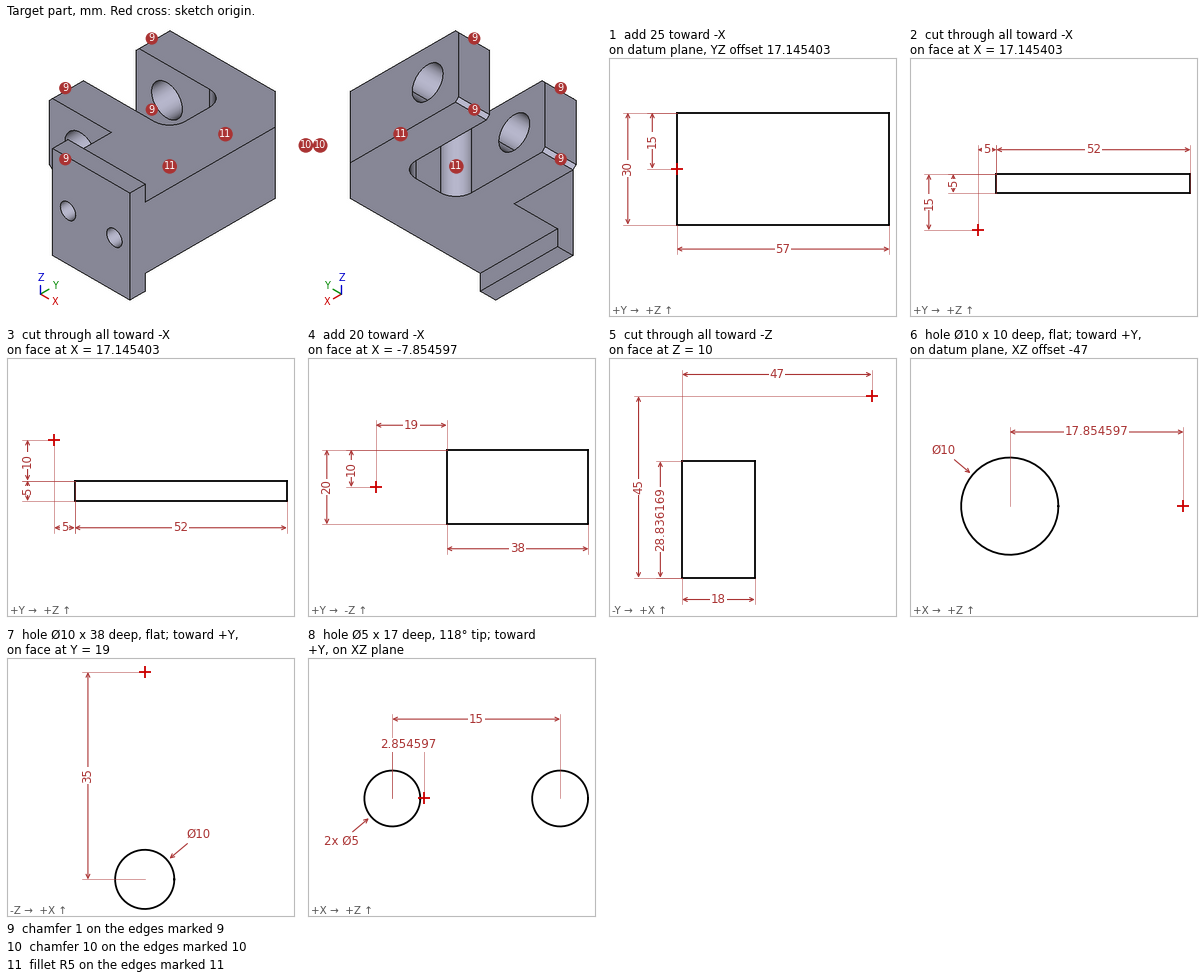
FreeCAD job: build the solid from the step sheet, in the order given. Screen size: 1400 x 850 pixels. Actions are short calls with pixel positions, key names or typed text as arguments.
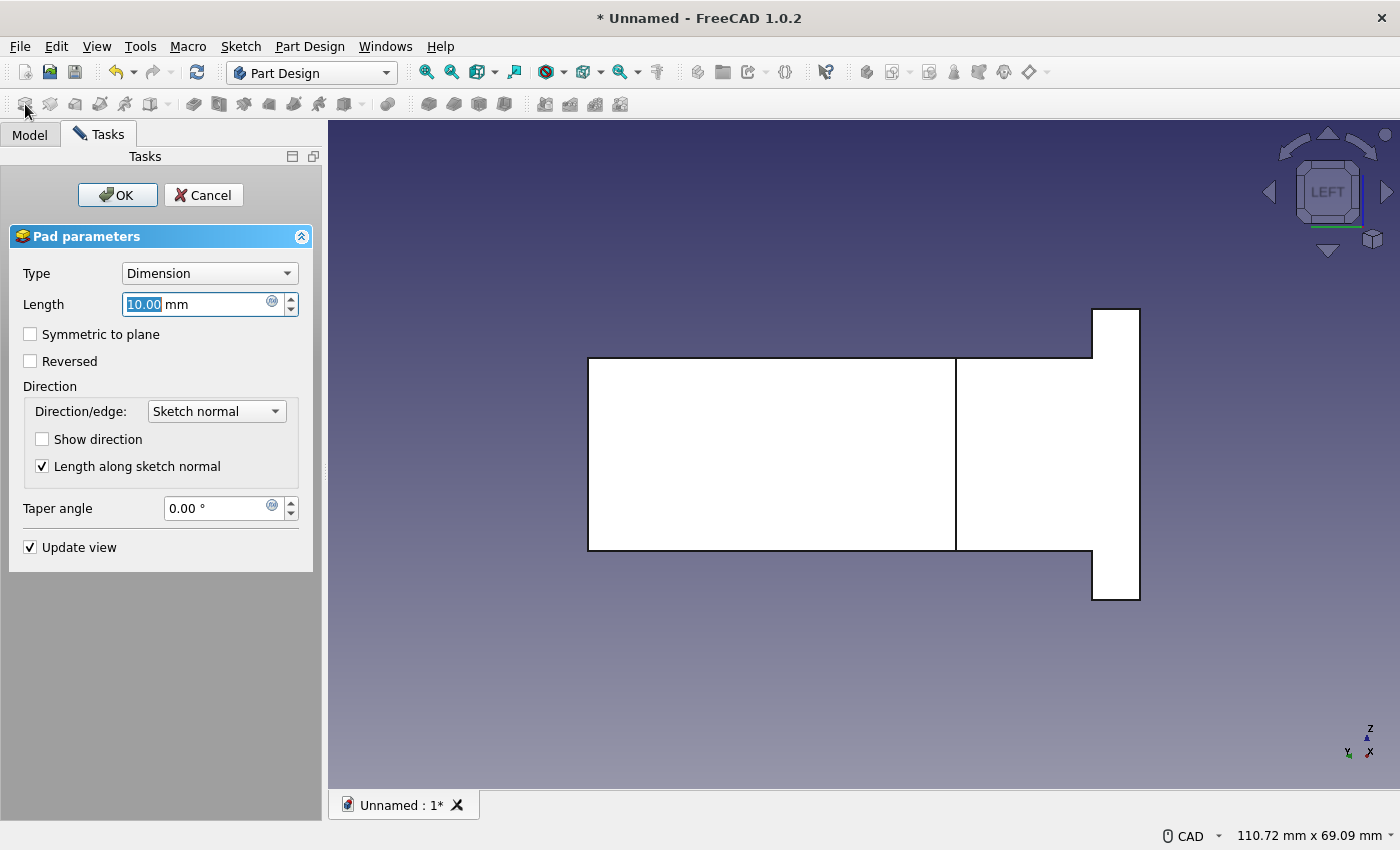
text(20)
key(Tab)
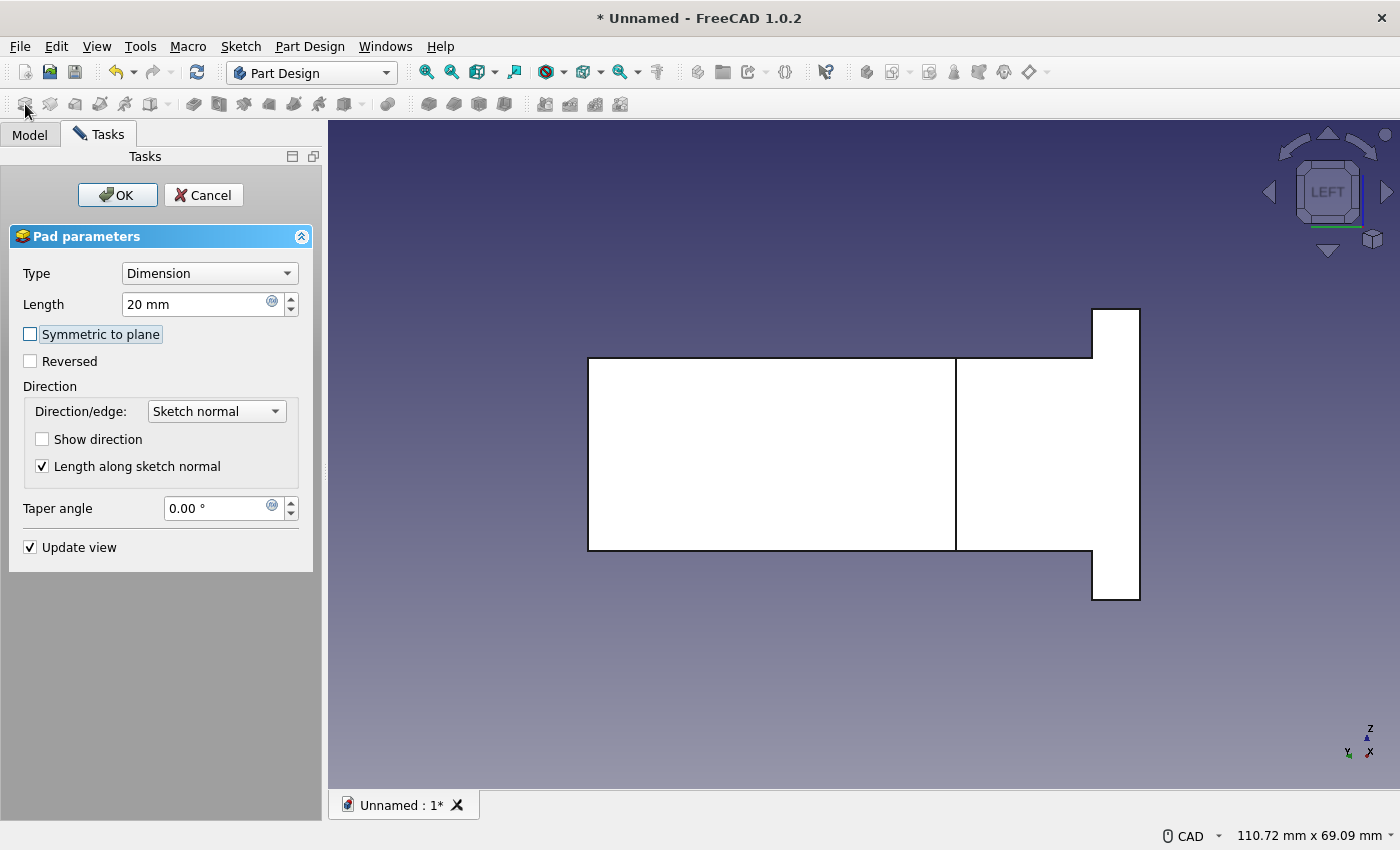
click(118, 195)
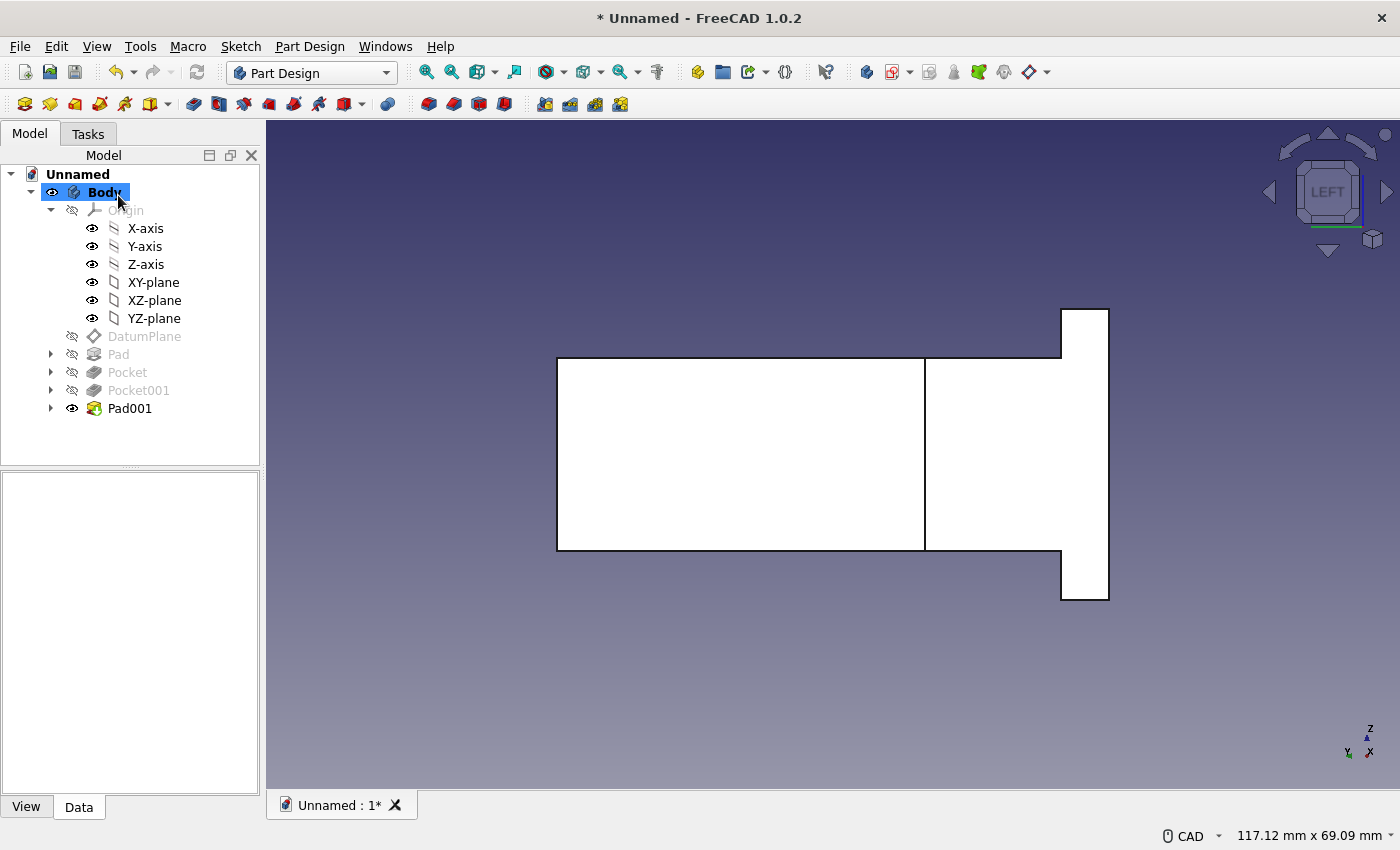
key(0)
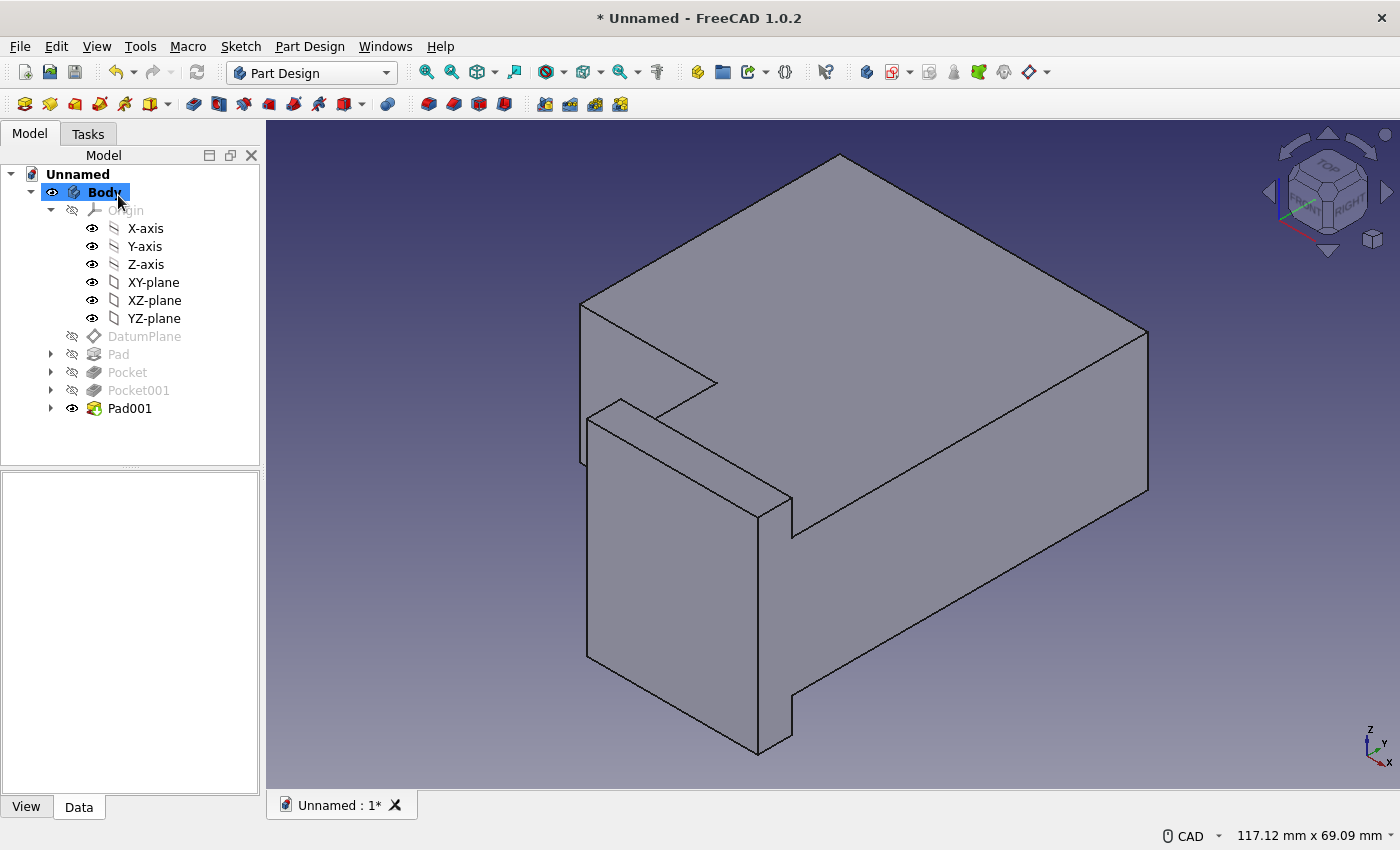
click(427, 72)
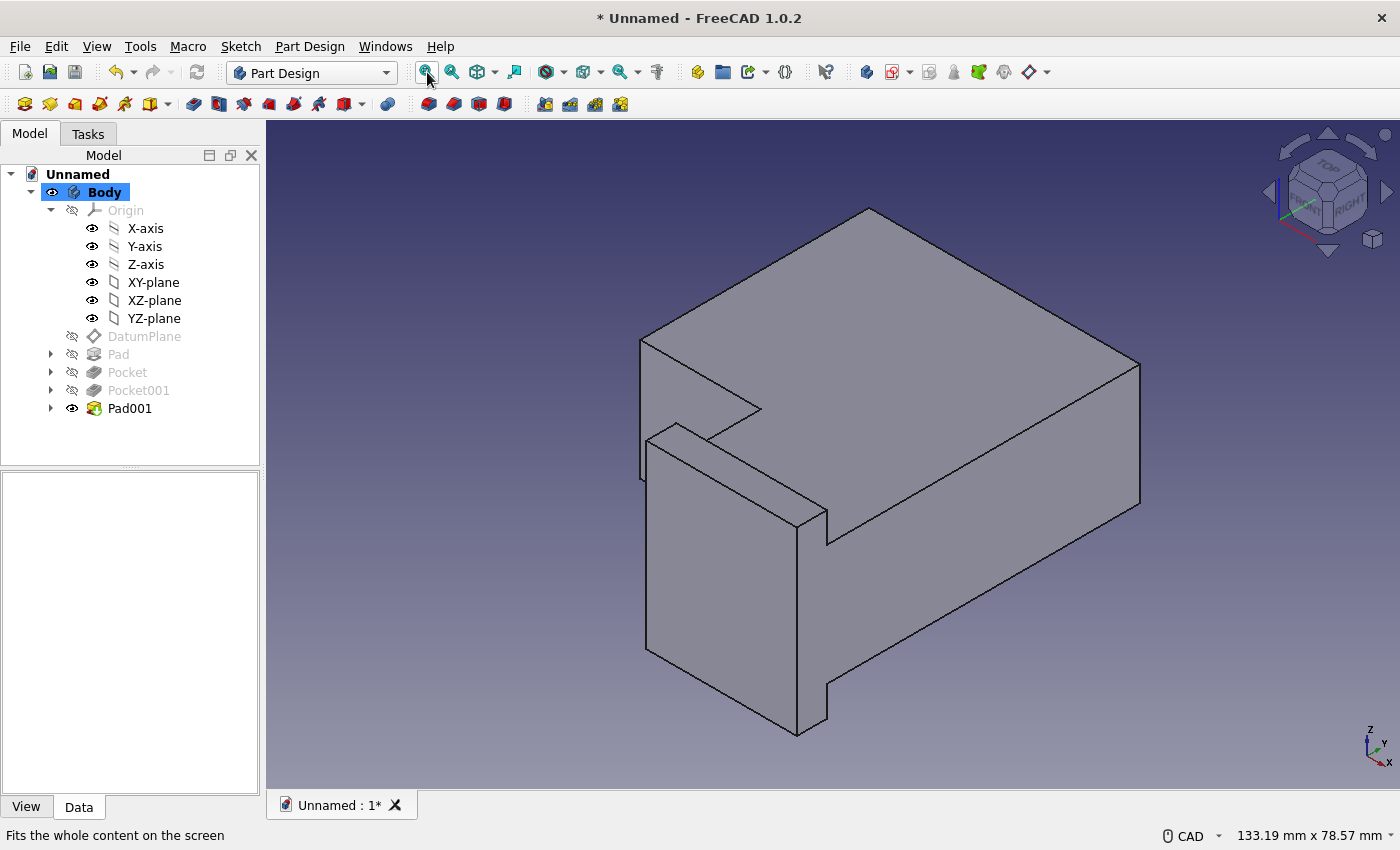
click(893, 349)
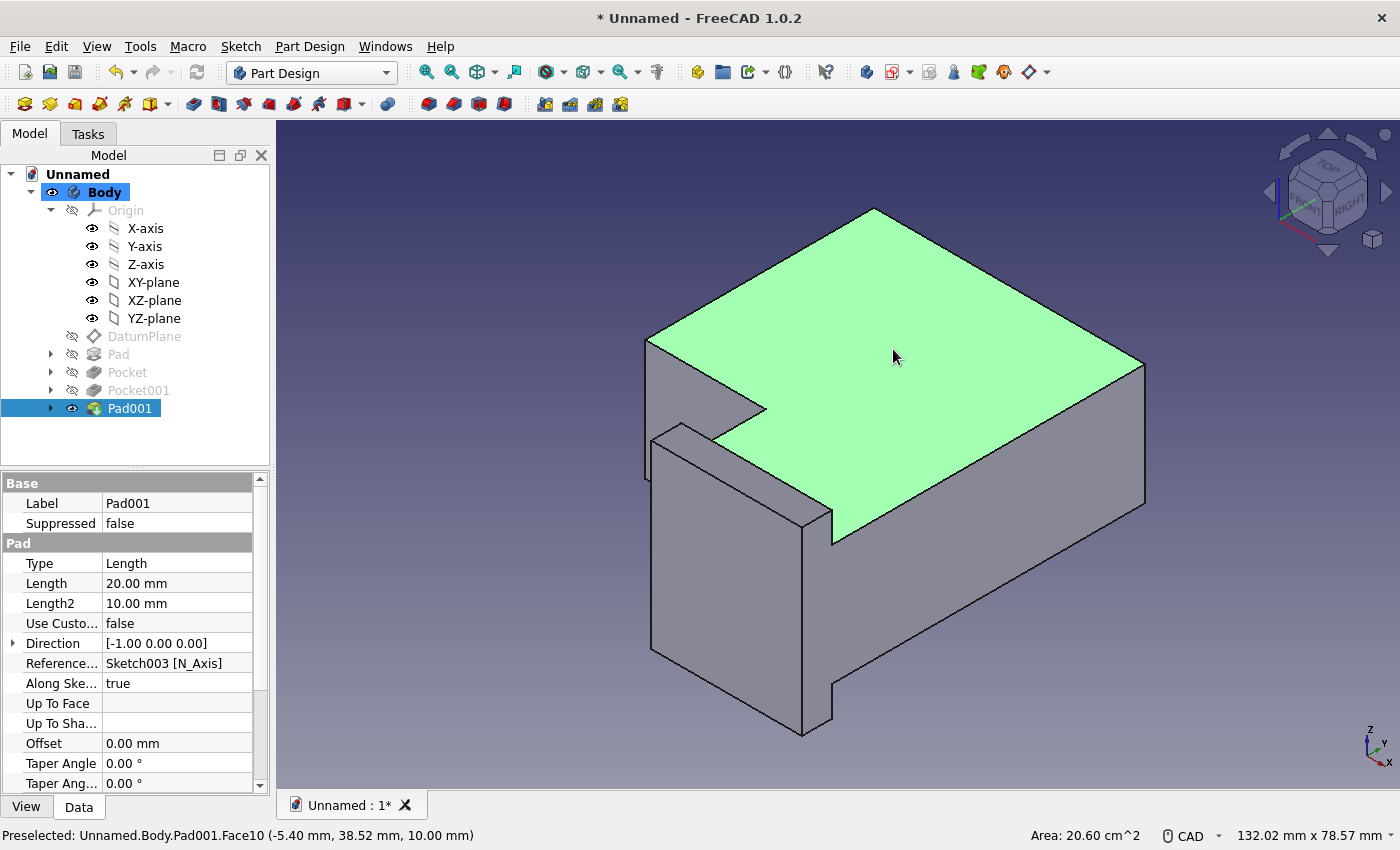
click(892, 72)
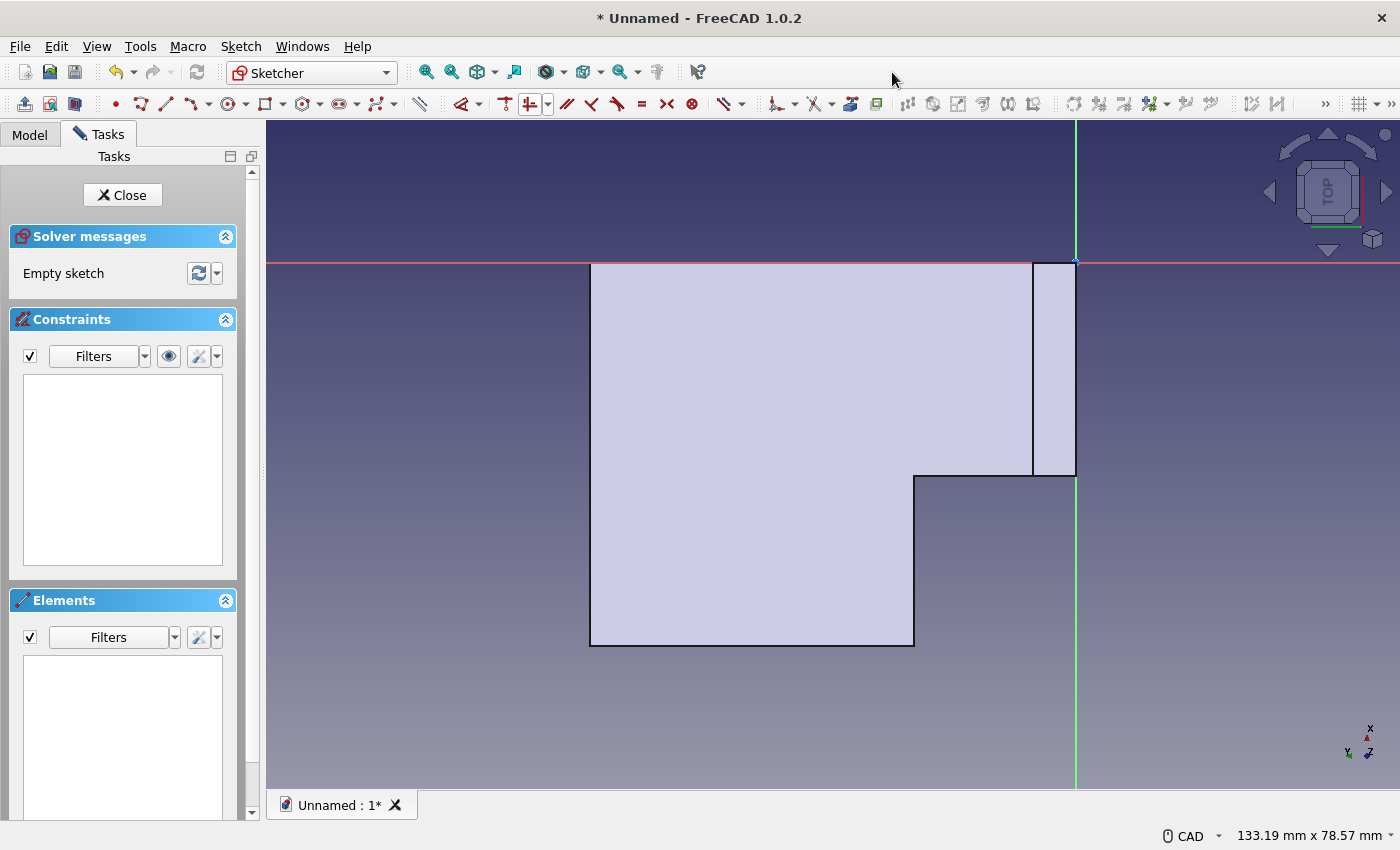
click(264, 104)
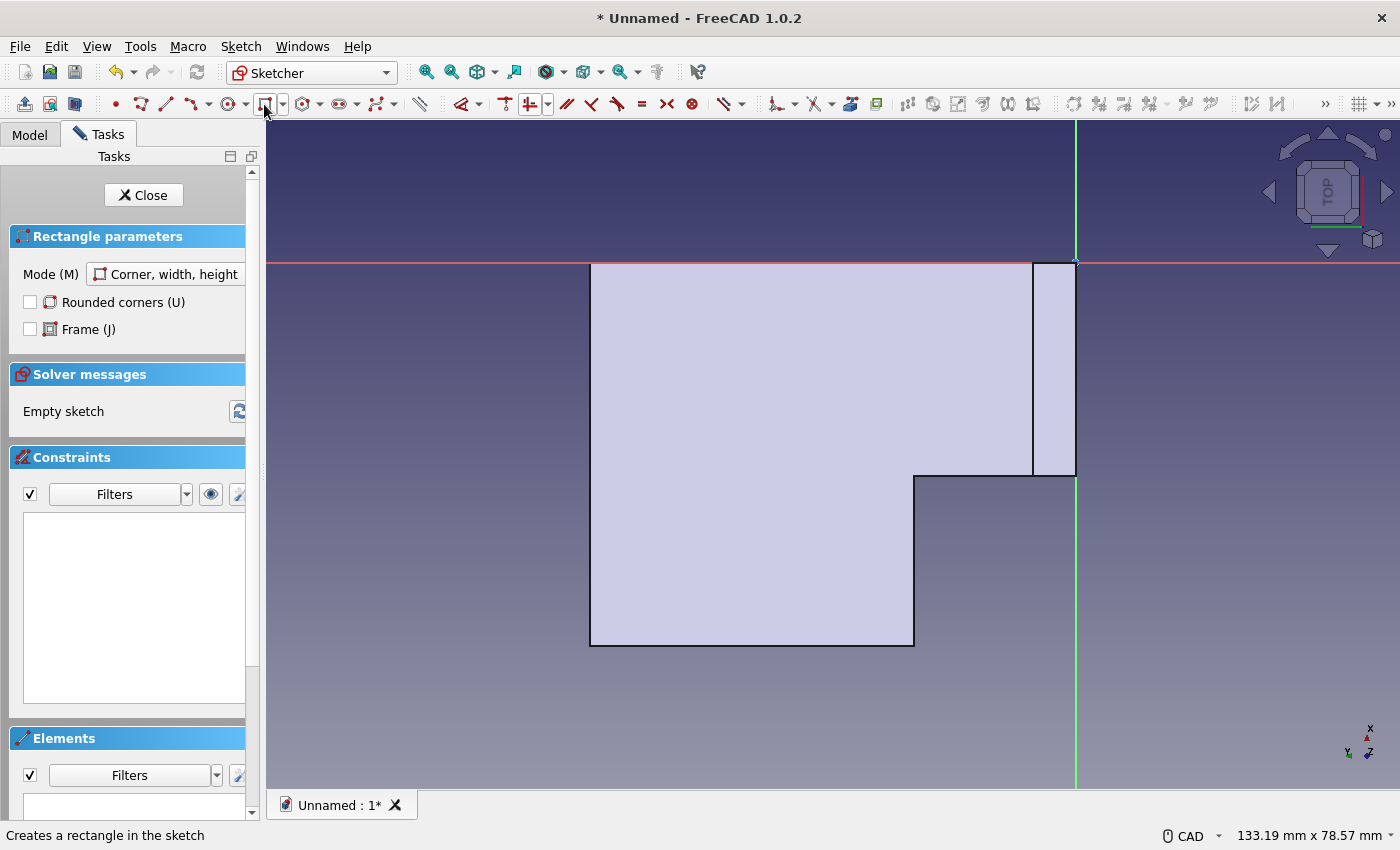
click(675, 401)
click(829, 646)
key(Escape)